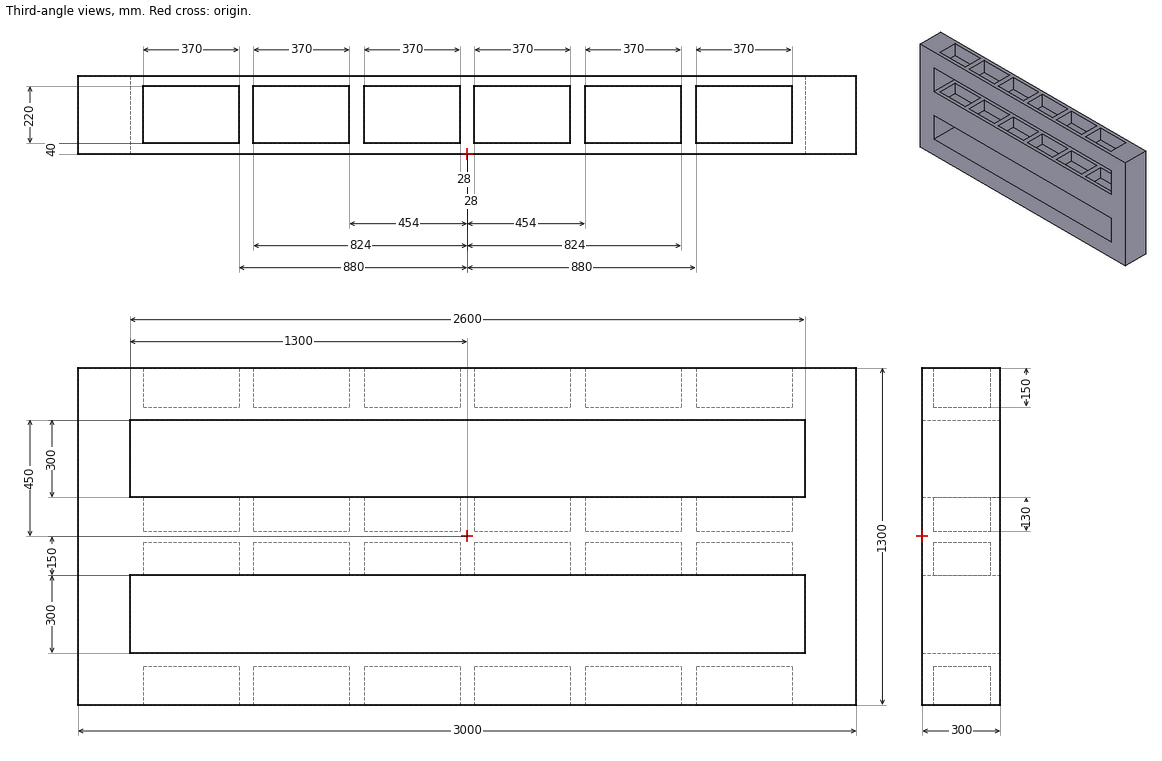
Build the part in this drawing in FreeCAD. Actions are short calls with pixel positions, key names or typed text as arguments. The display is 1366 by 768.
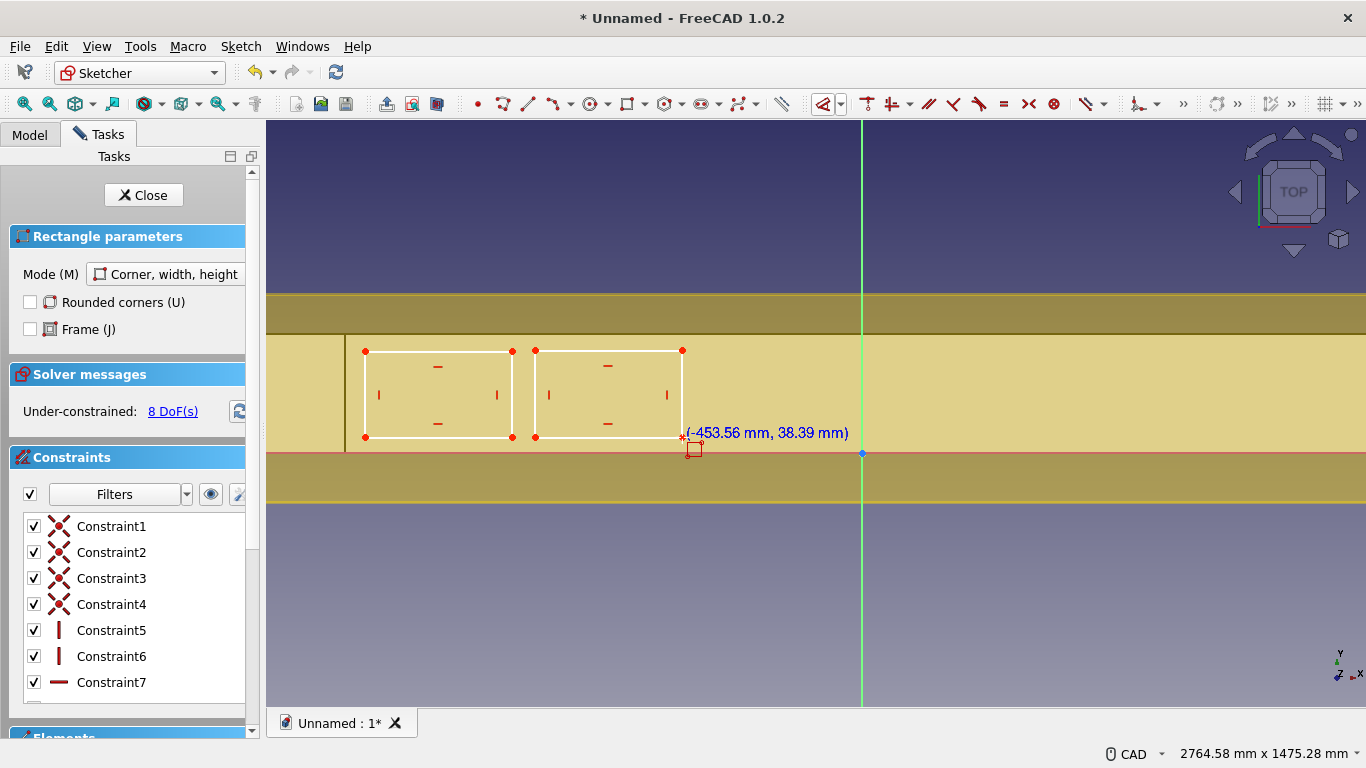
click(704, 350)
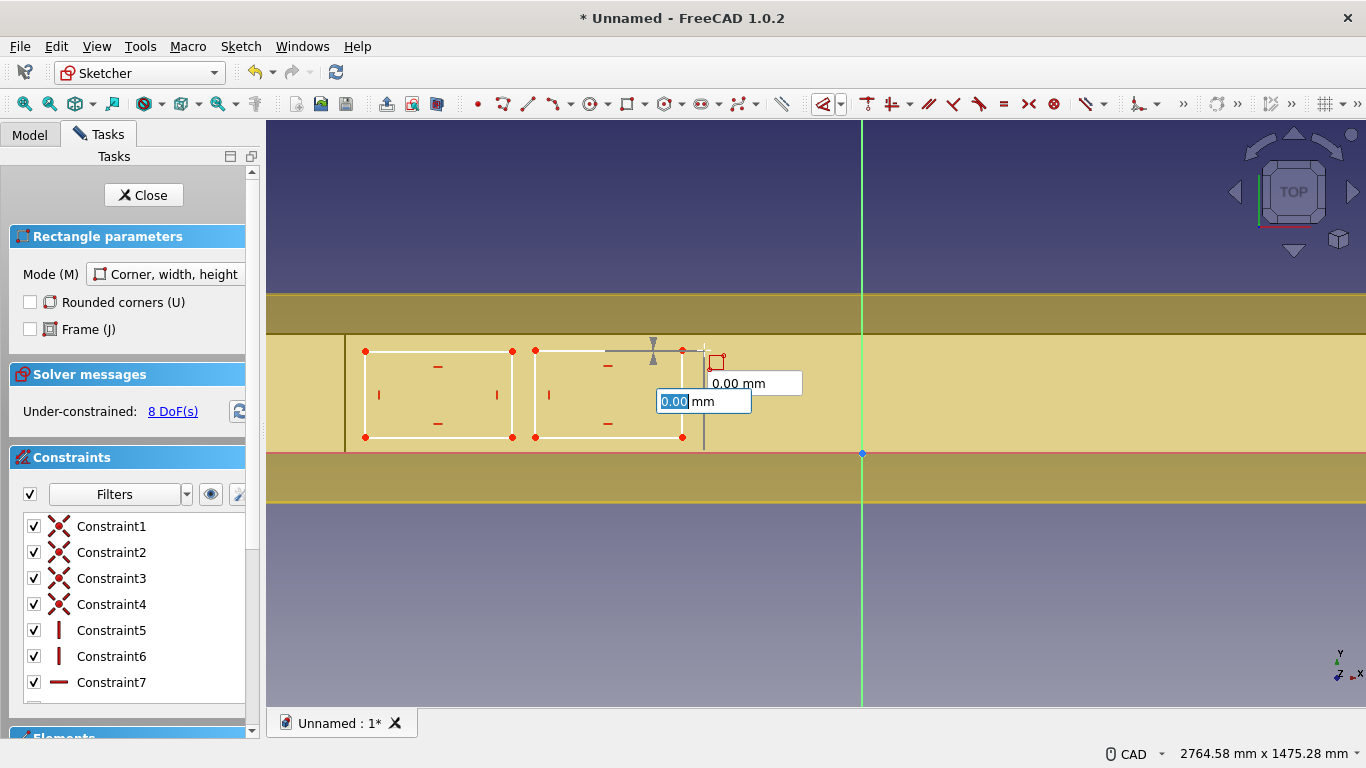
scroll(851, 437, up, 2)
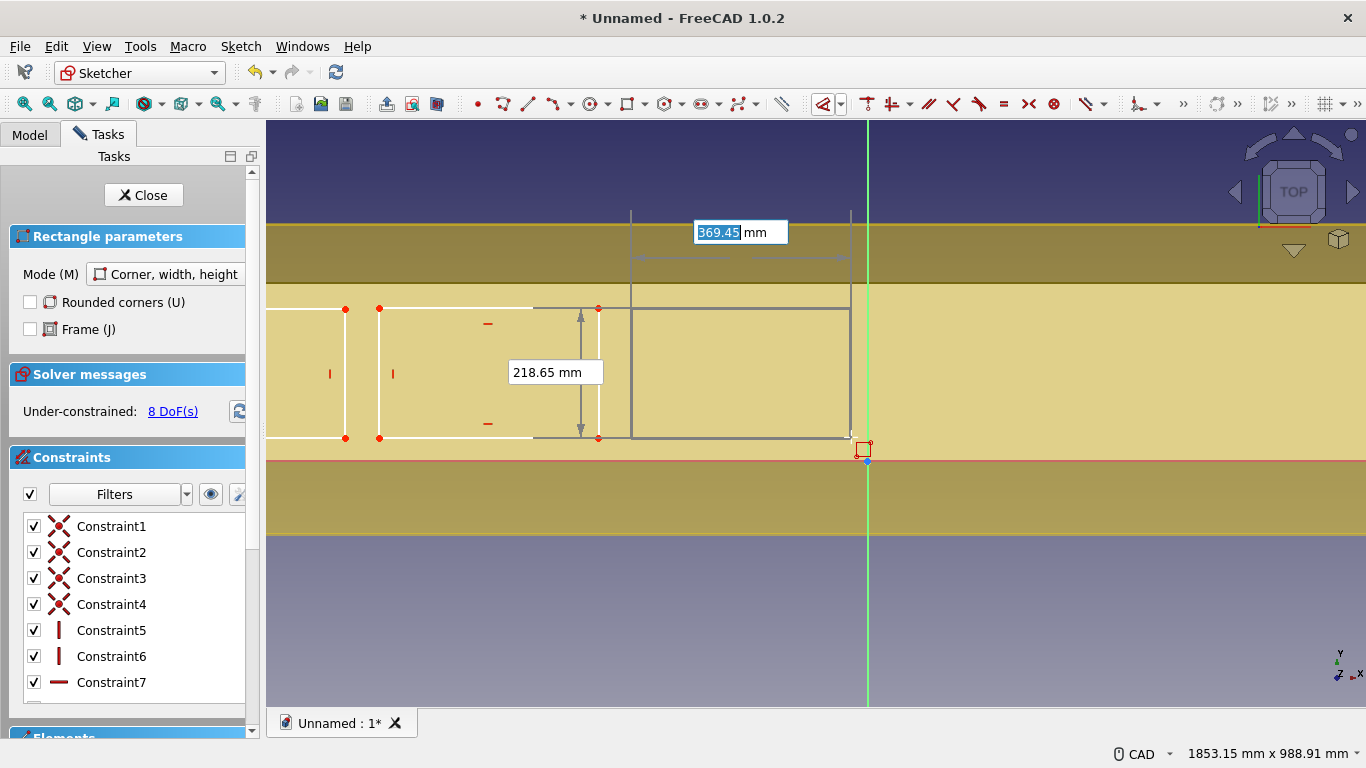
click(851, 437)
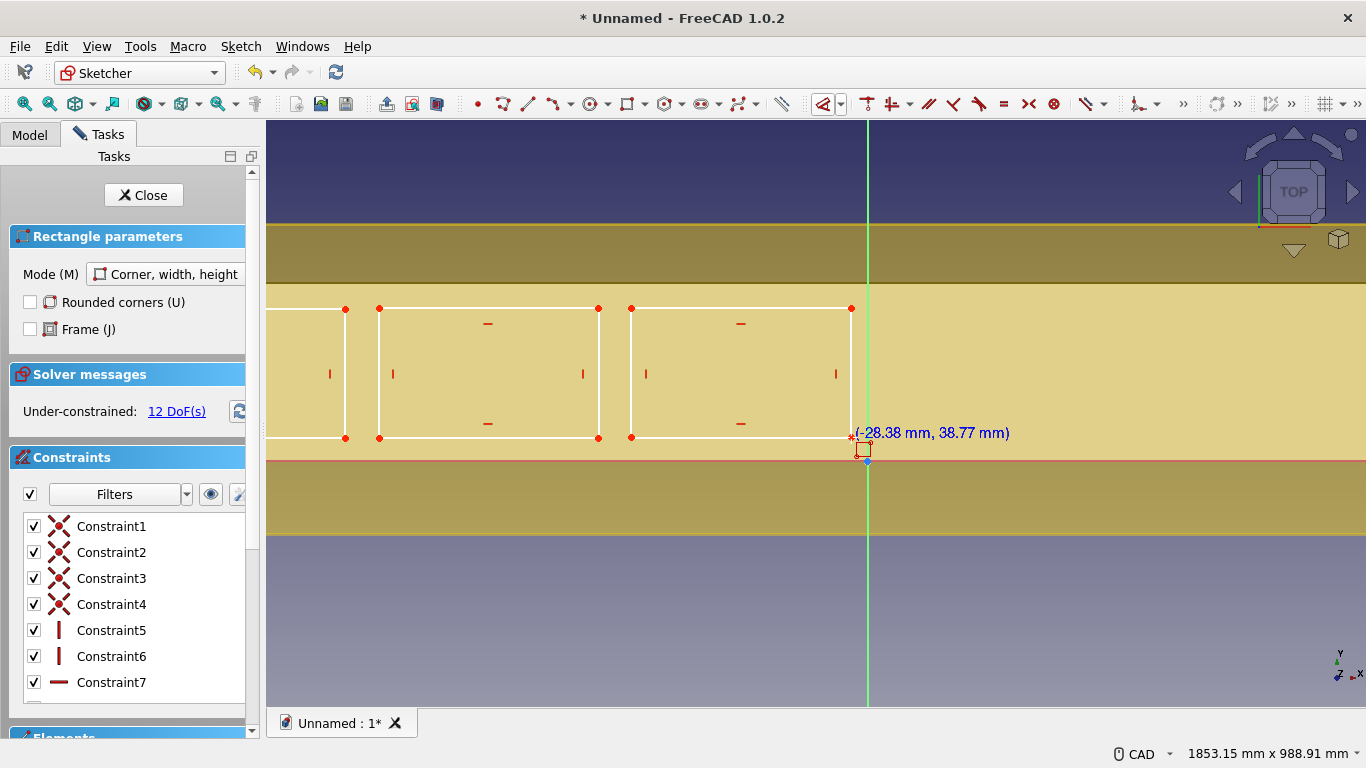
click(884, 307)
click(1104, 437)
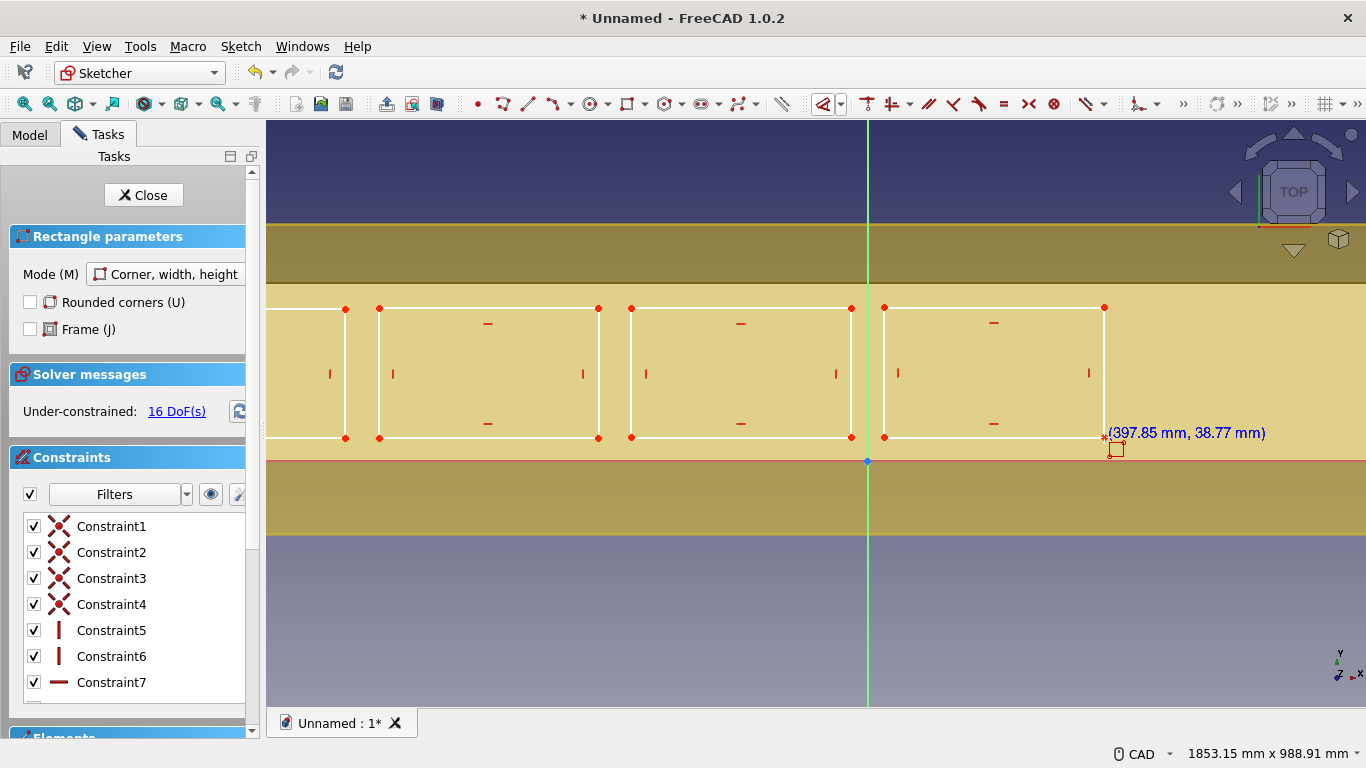
click(1137, 307)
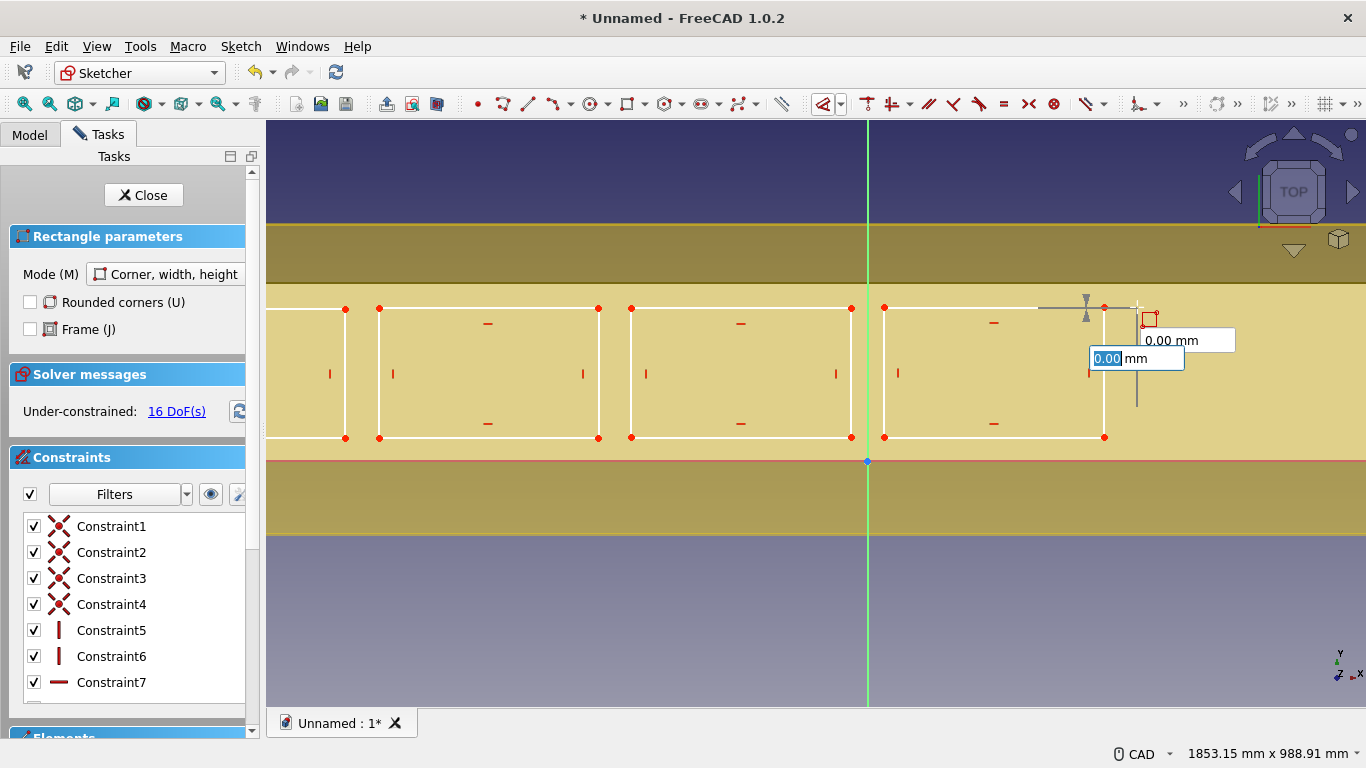
scroll(649, 438, down, 4)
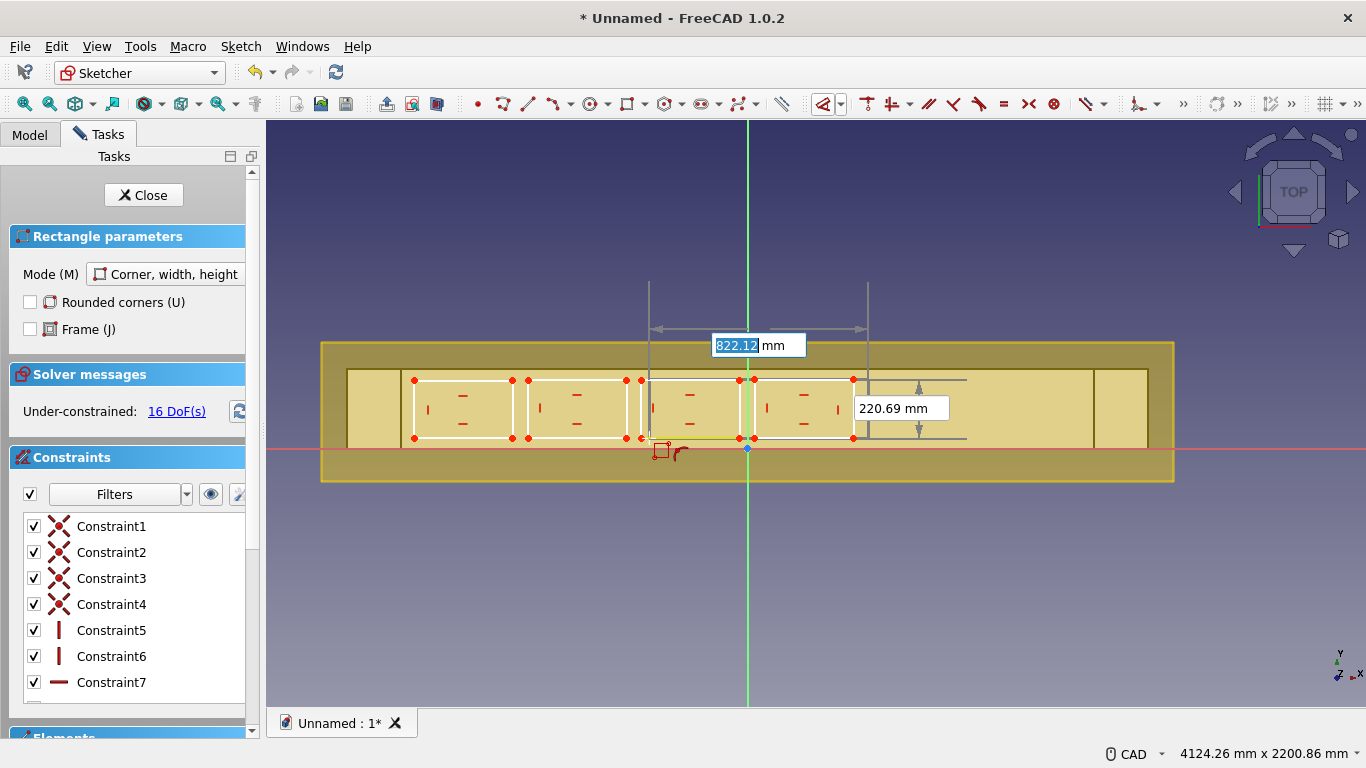
scroll(967, 438, up, 2)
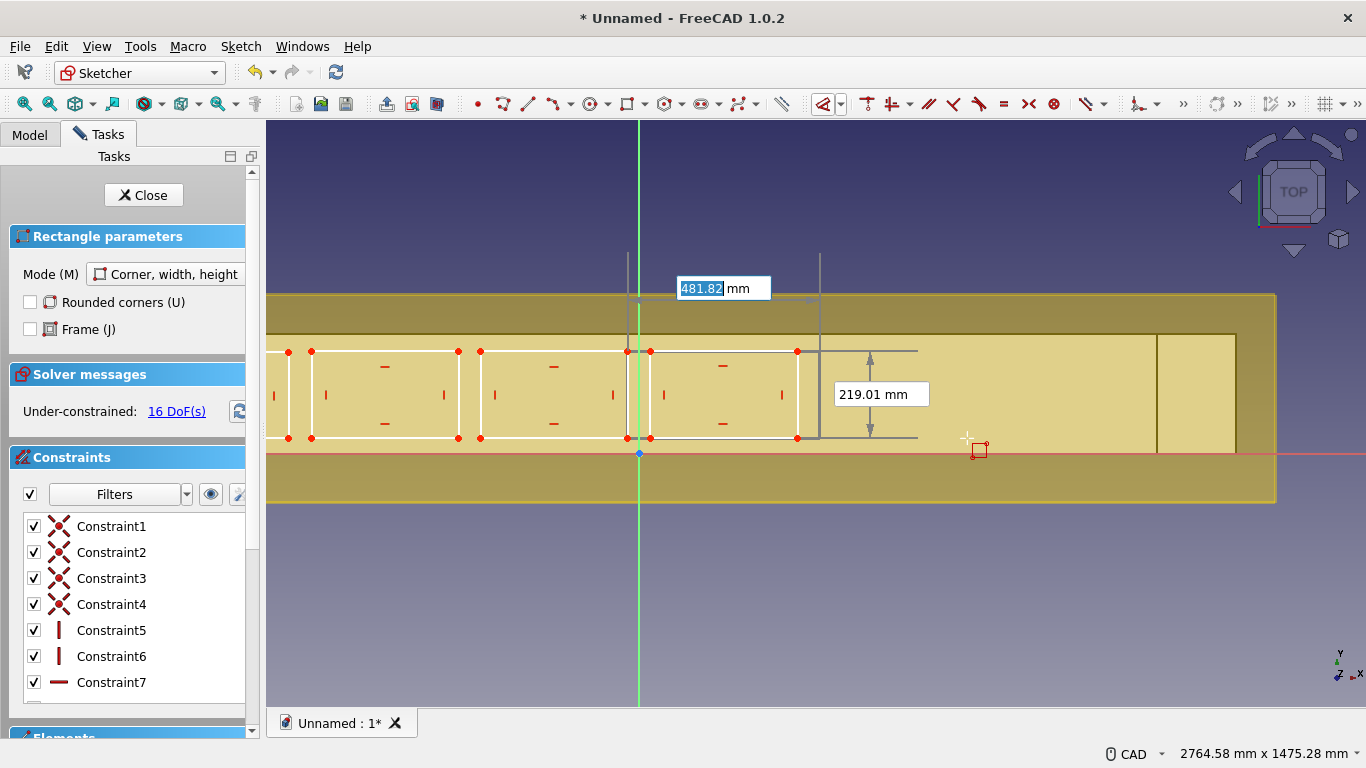
click(967, 438)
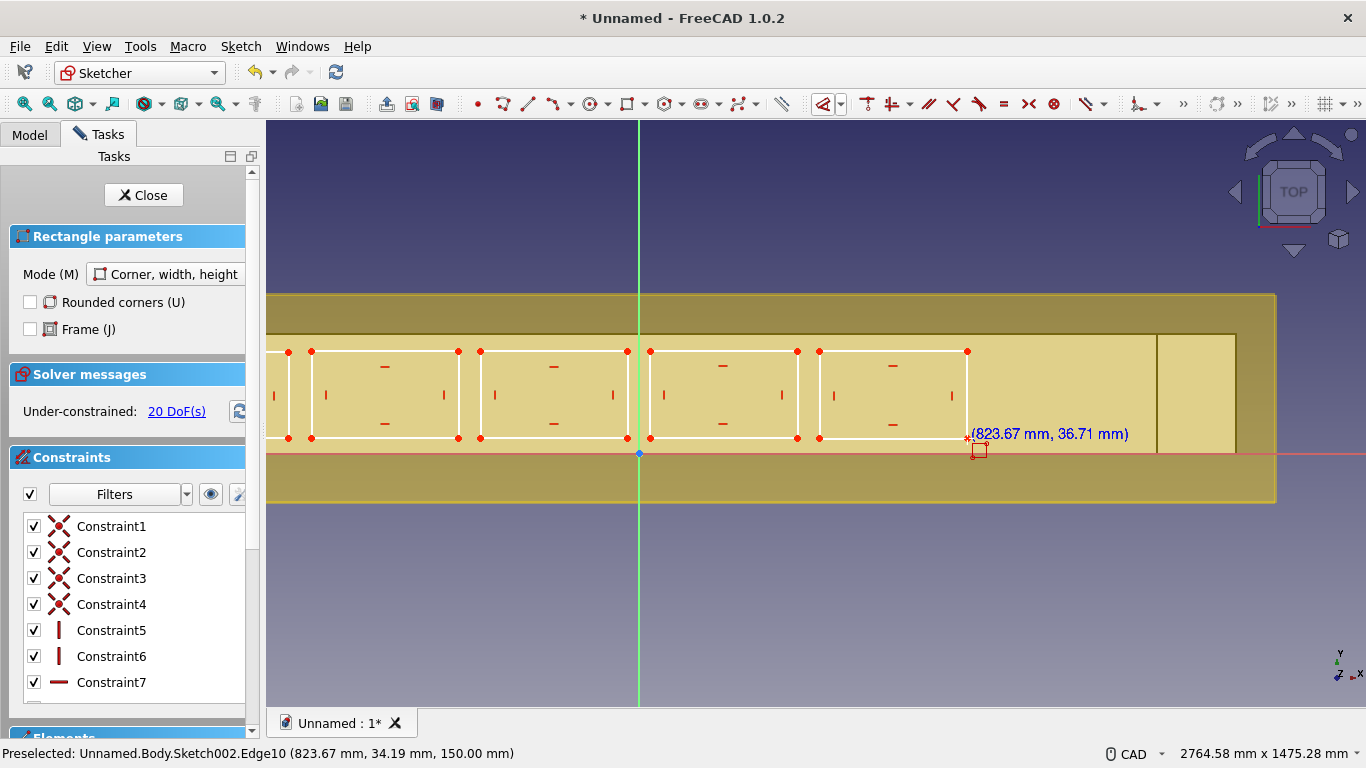
click(989, 350)
click(1137, 438)
key(Escape)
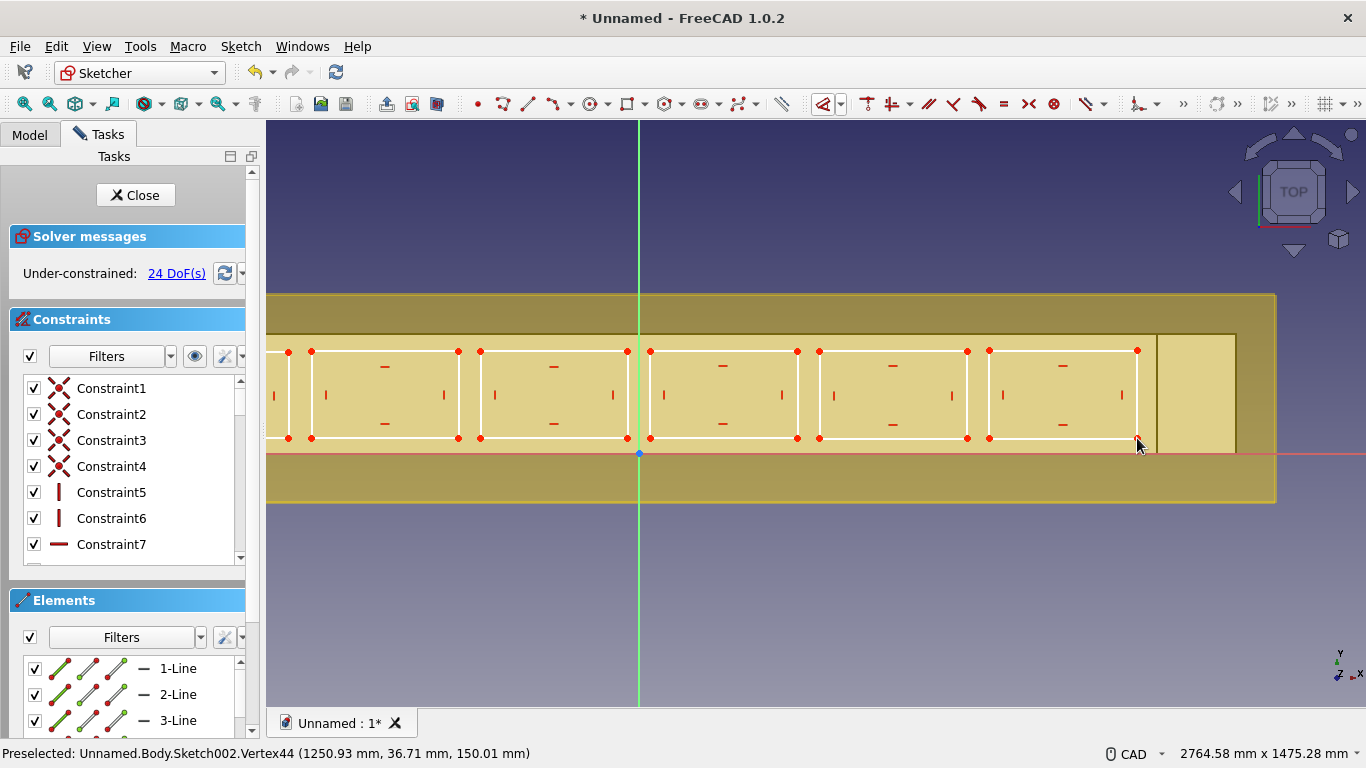
scroll(968, 437, down, 2)